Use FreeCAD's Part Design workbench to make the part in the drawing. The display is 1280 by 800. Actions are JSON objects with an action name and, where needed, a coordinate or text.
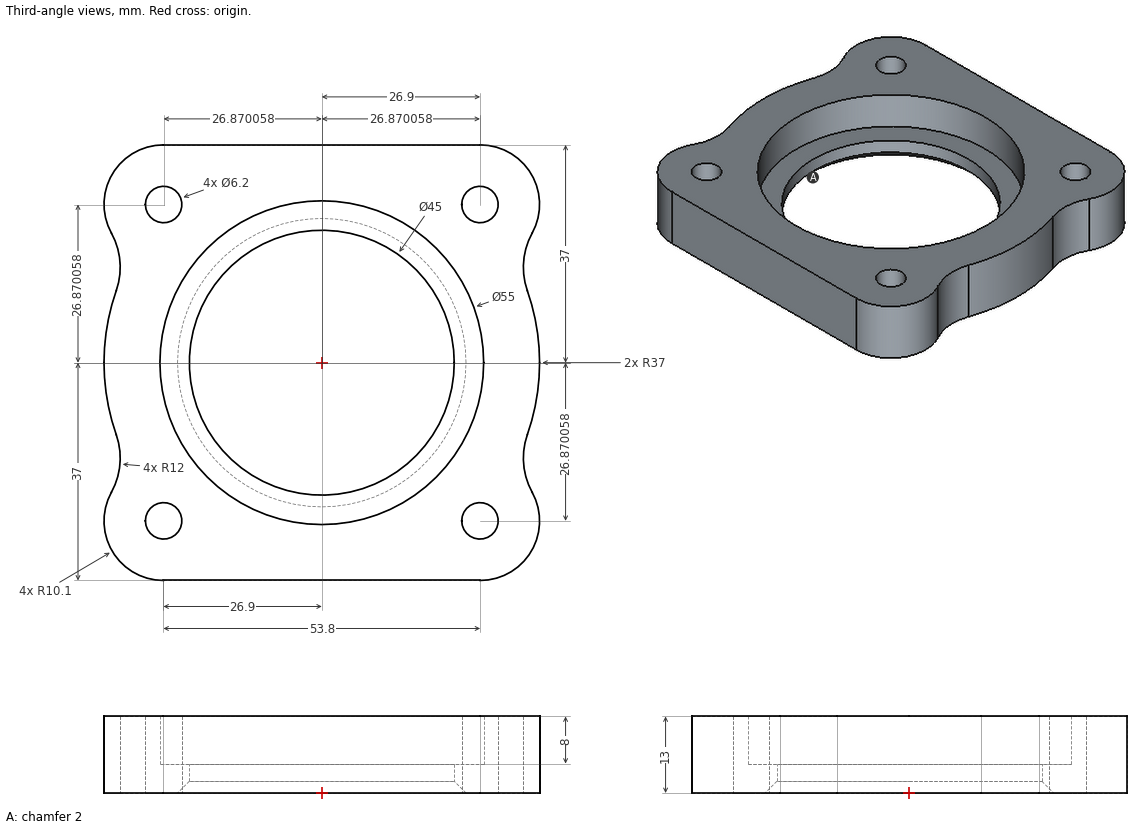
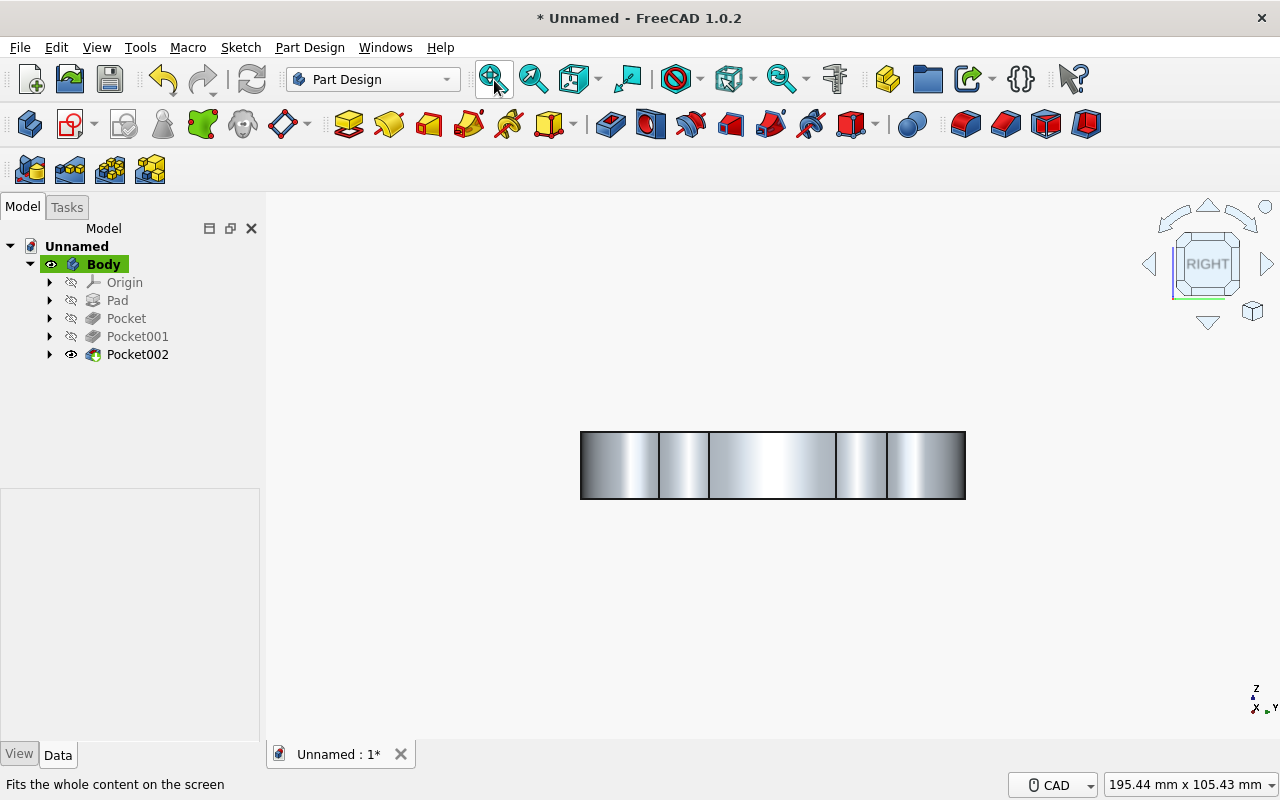
{"action": "key", "text": "5"}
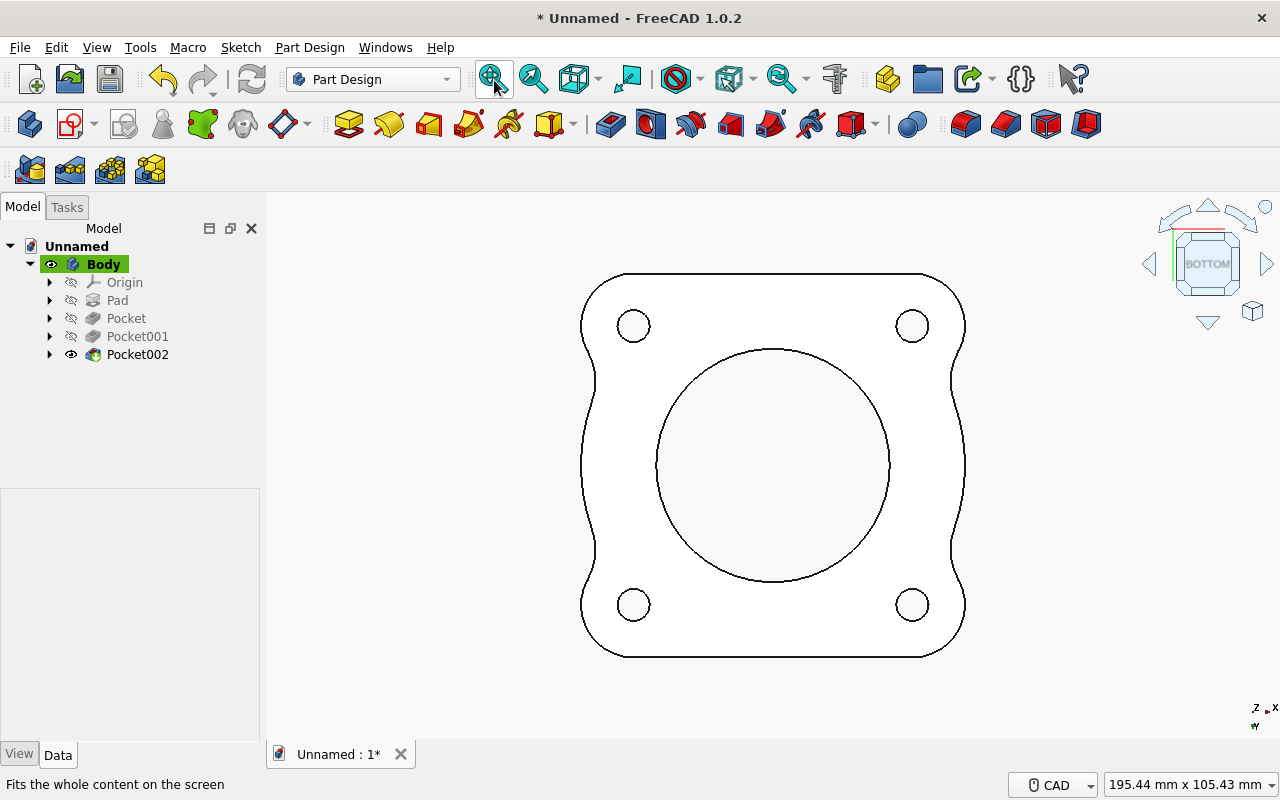
{"action": "left_click", "coordinate": [656, 464]}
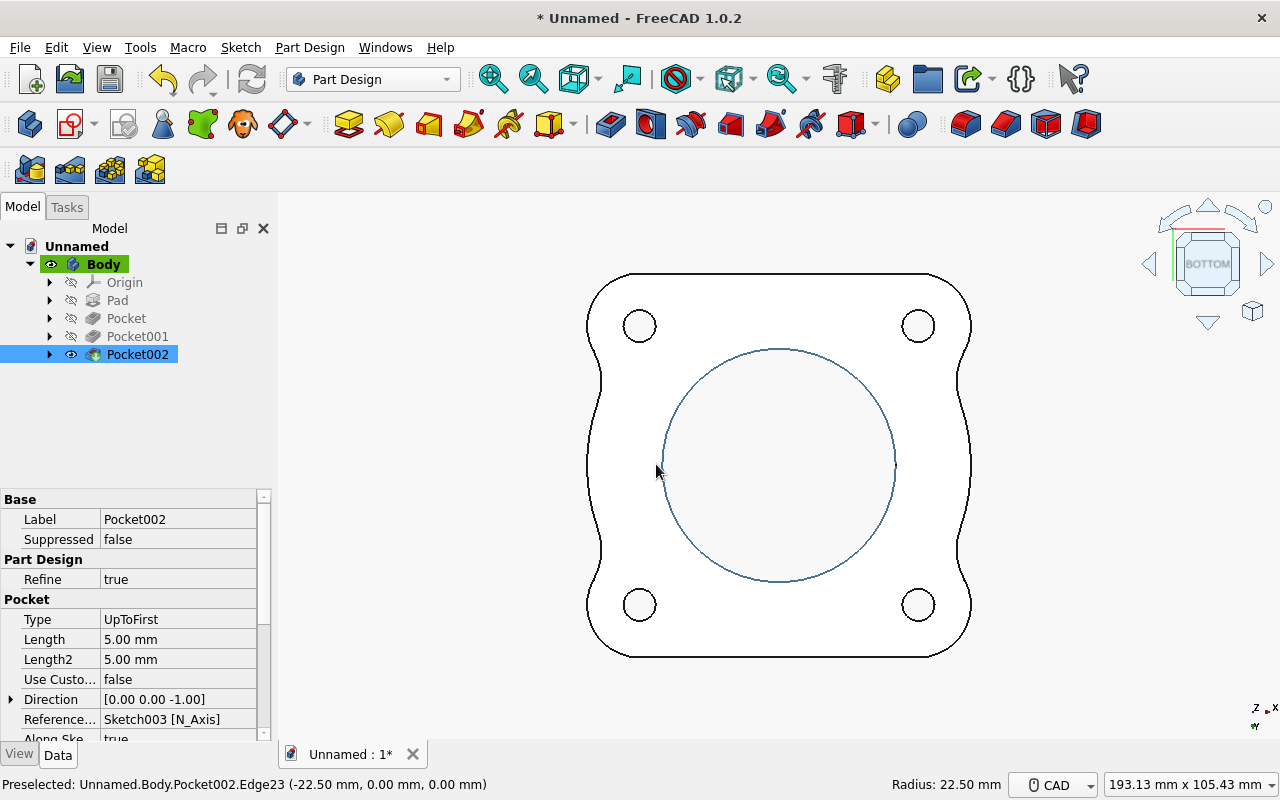
{"action": "left_click", "coordinate": [1006, 124]}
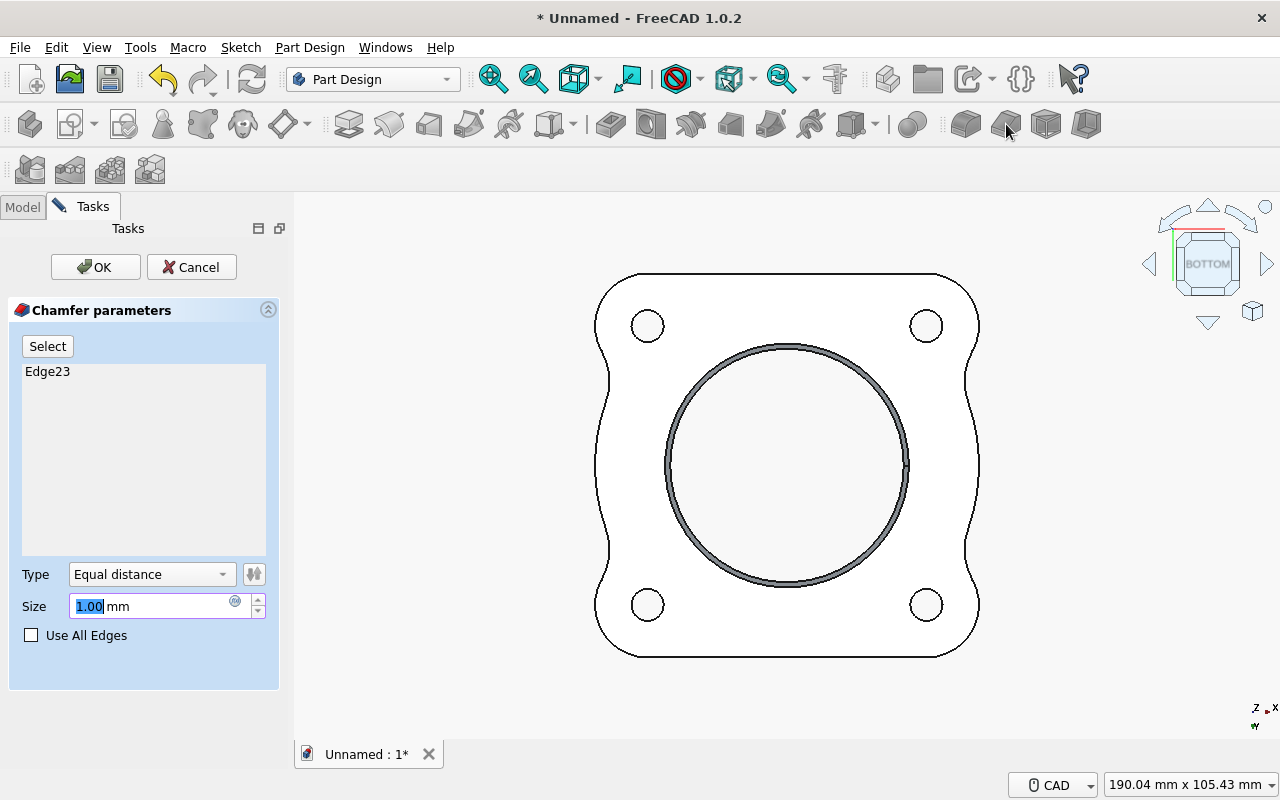
{"action": "type", "text": "2"}
{"action": "key", "text": "Tab"}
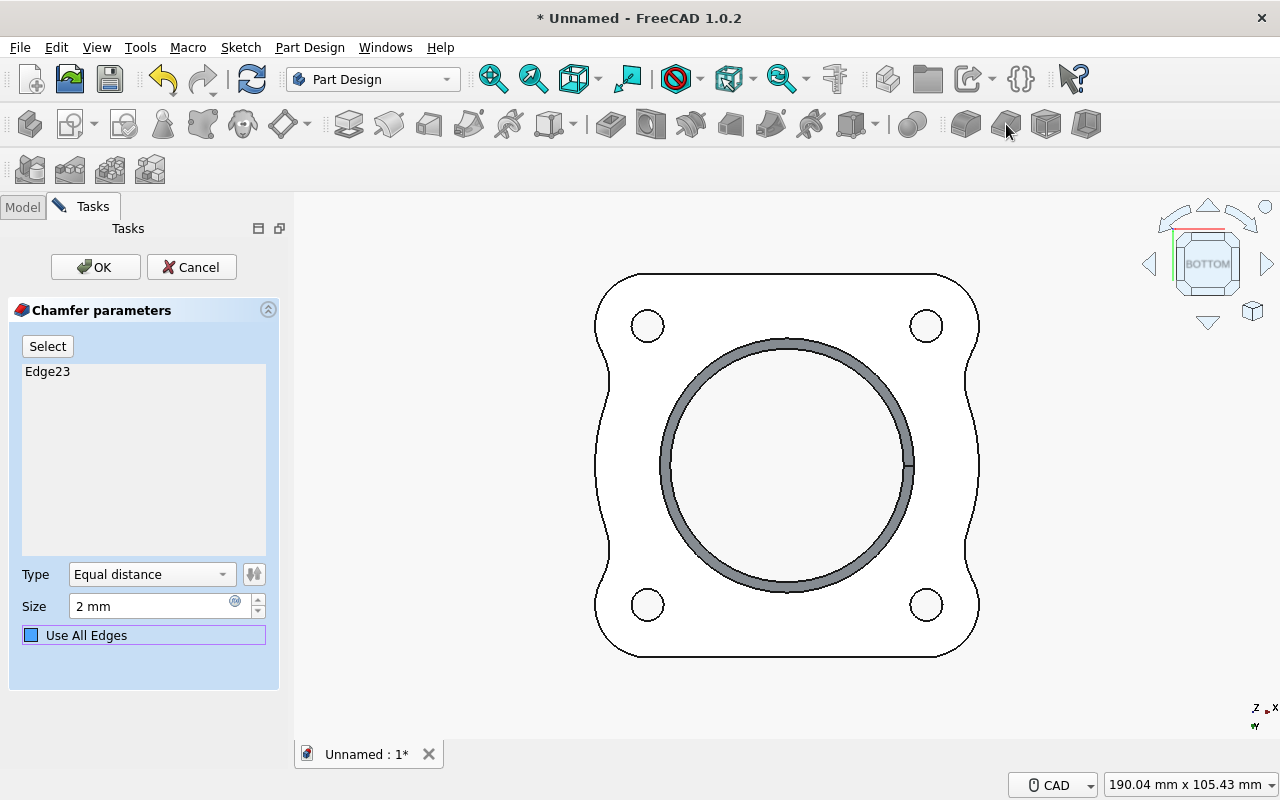
{"action": "left_click", "coordinate": [96, 267]}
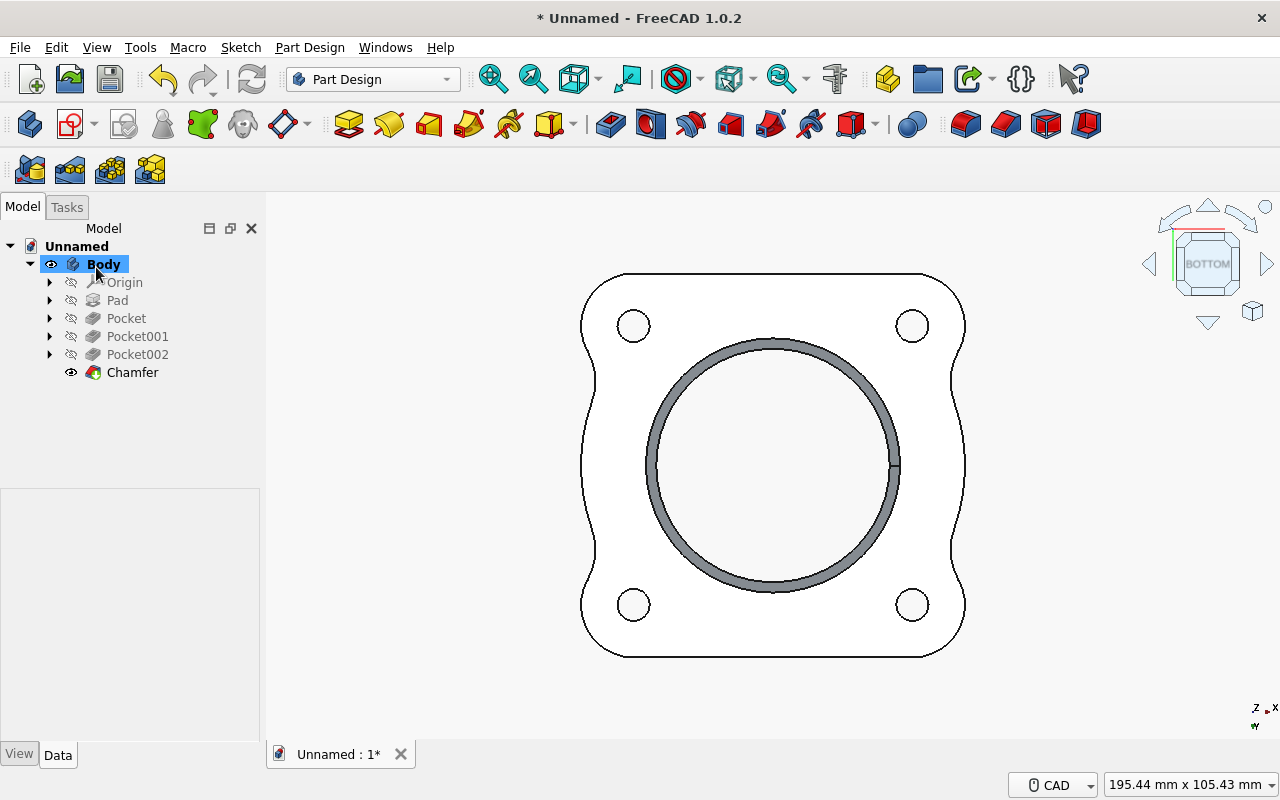
{"action": "key", "text": "0"}